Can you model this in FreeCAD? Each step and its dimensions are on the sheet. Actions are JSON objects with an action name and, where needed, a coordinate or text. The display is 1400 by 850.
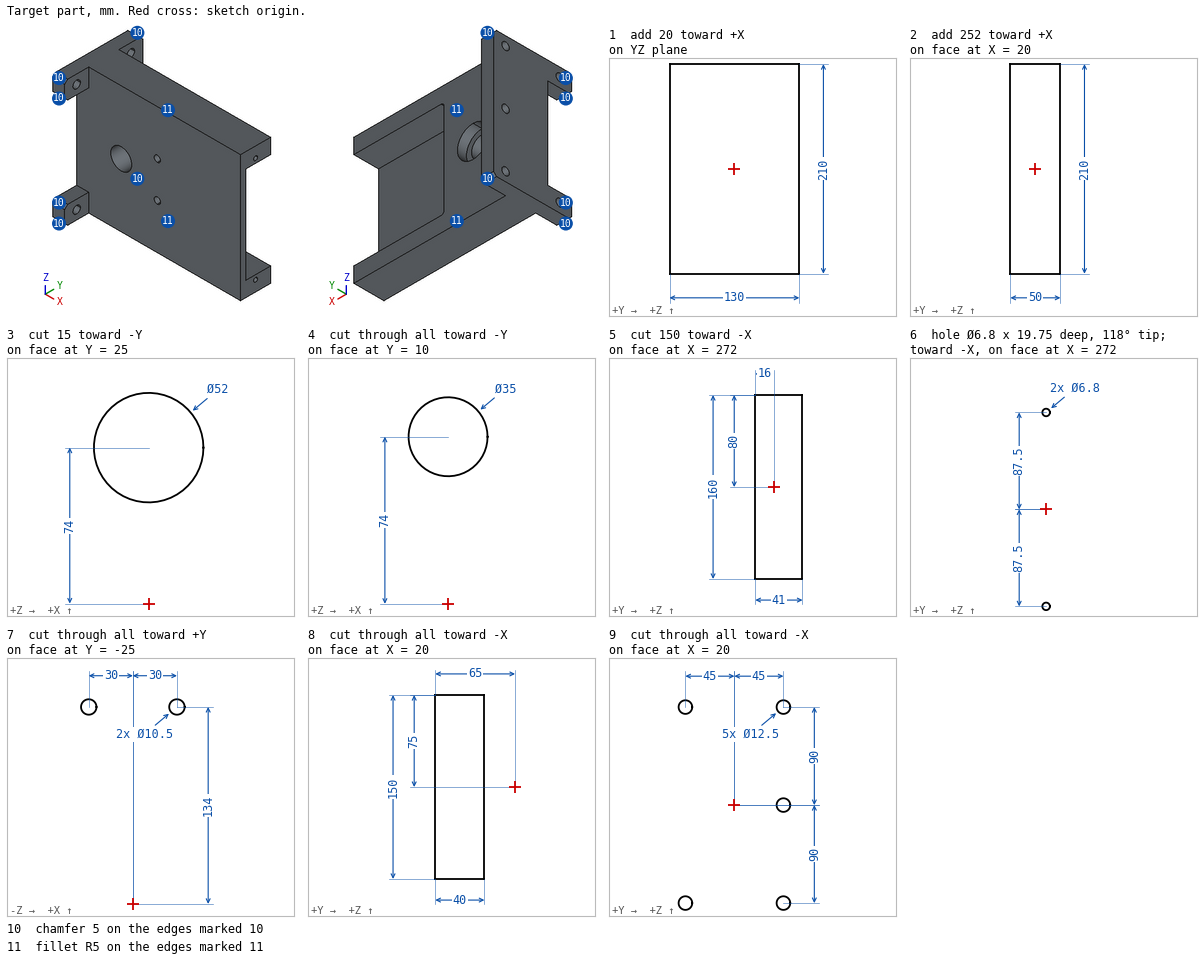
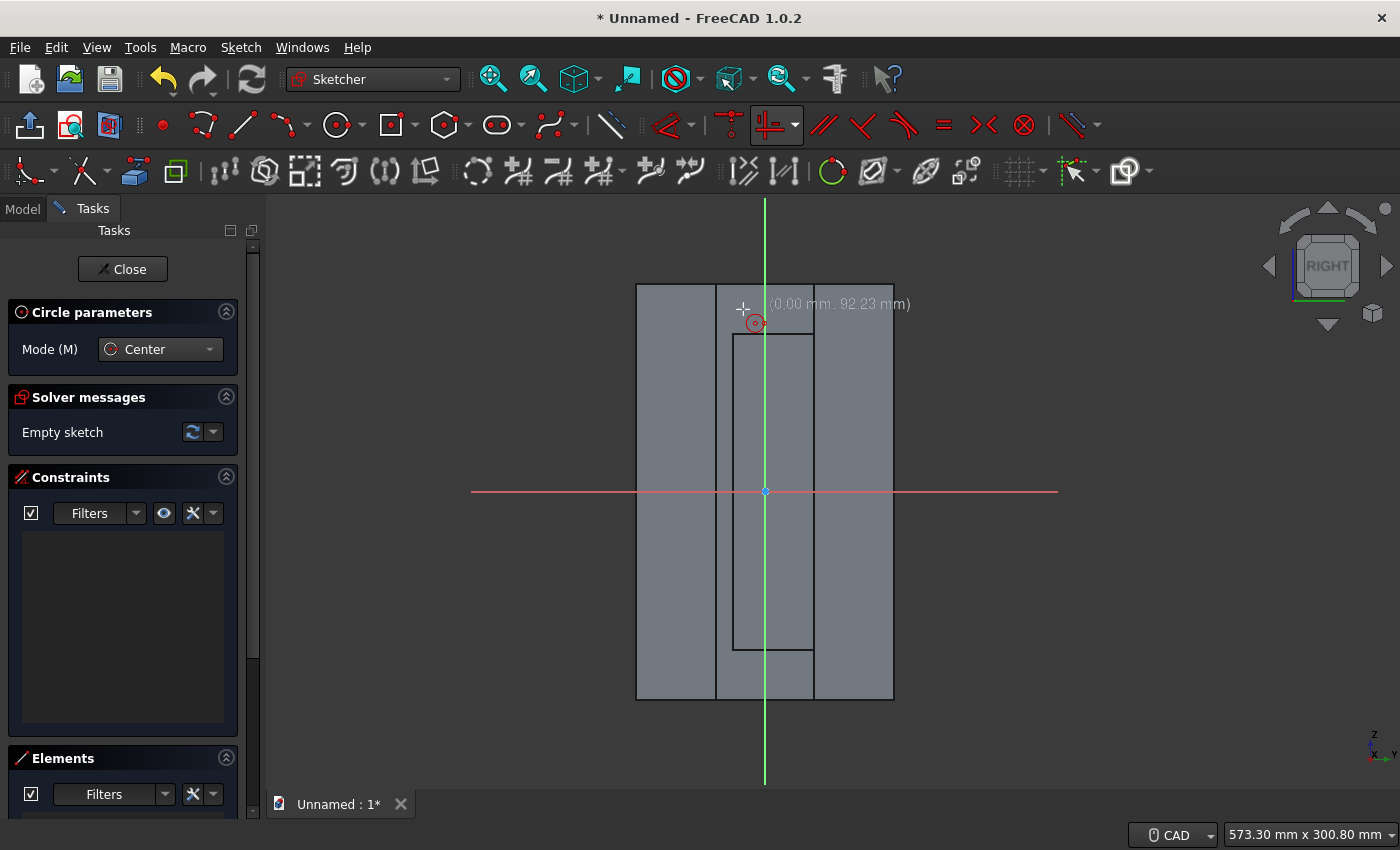
{"action": "left_click", "coordinate": [765, 319]}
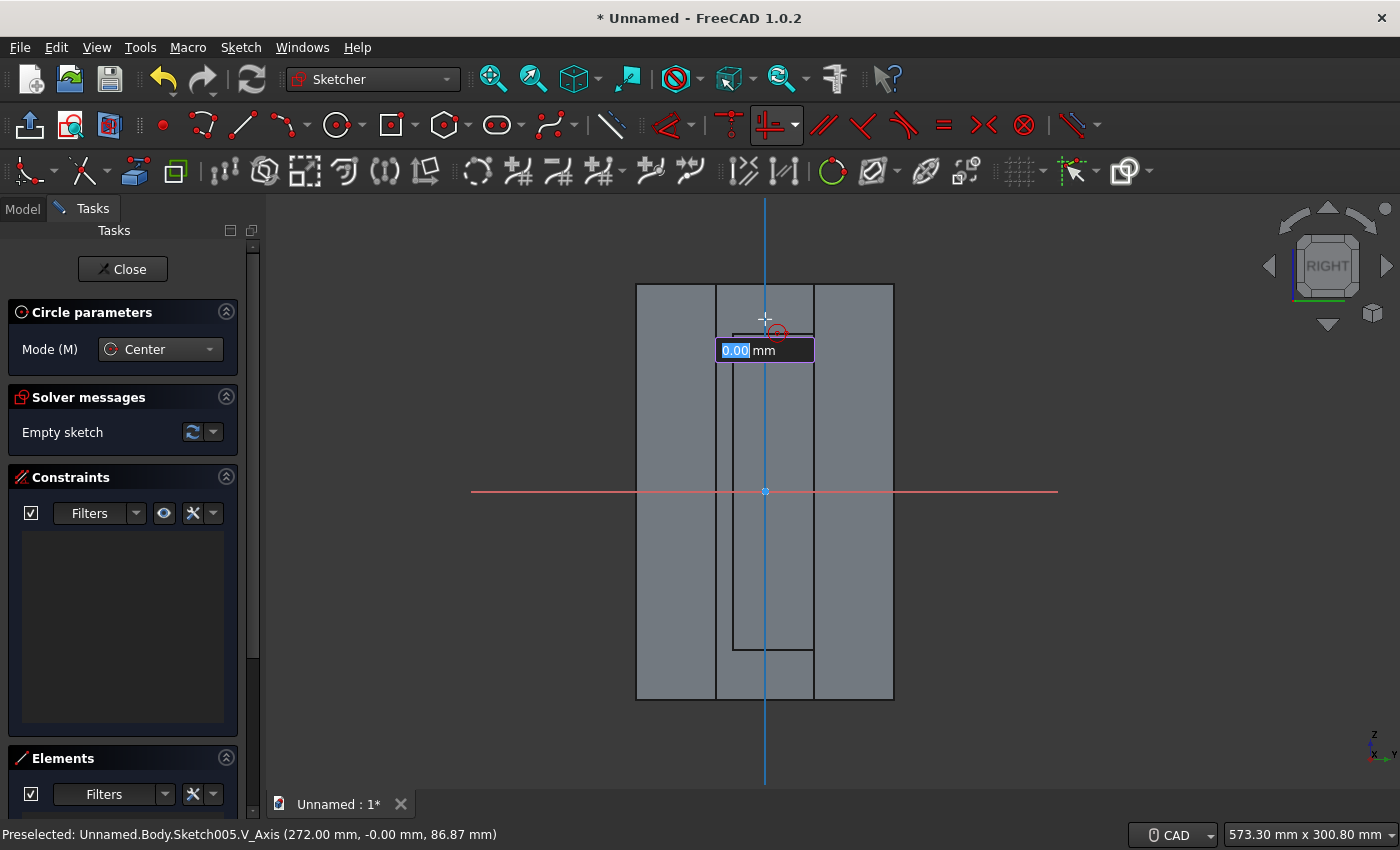
{"action": "scroll", "coordinate": [771, 316], "scroll_direction": "up", "scroll_amount": 5}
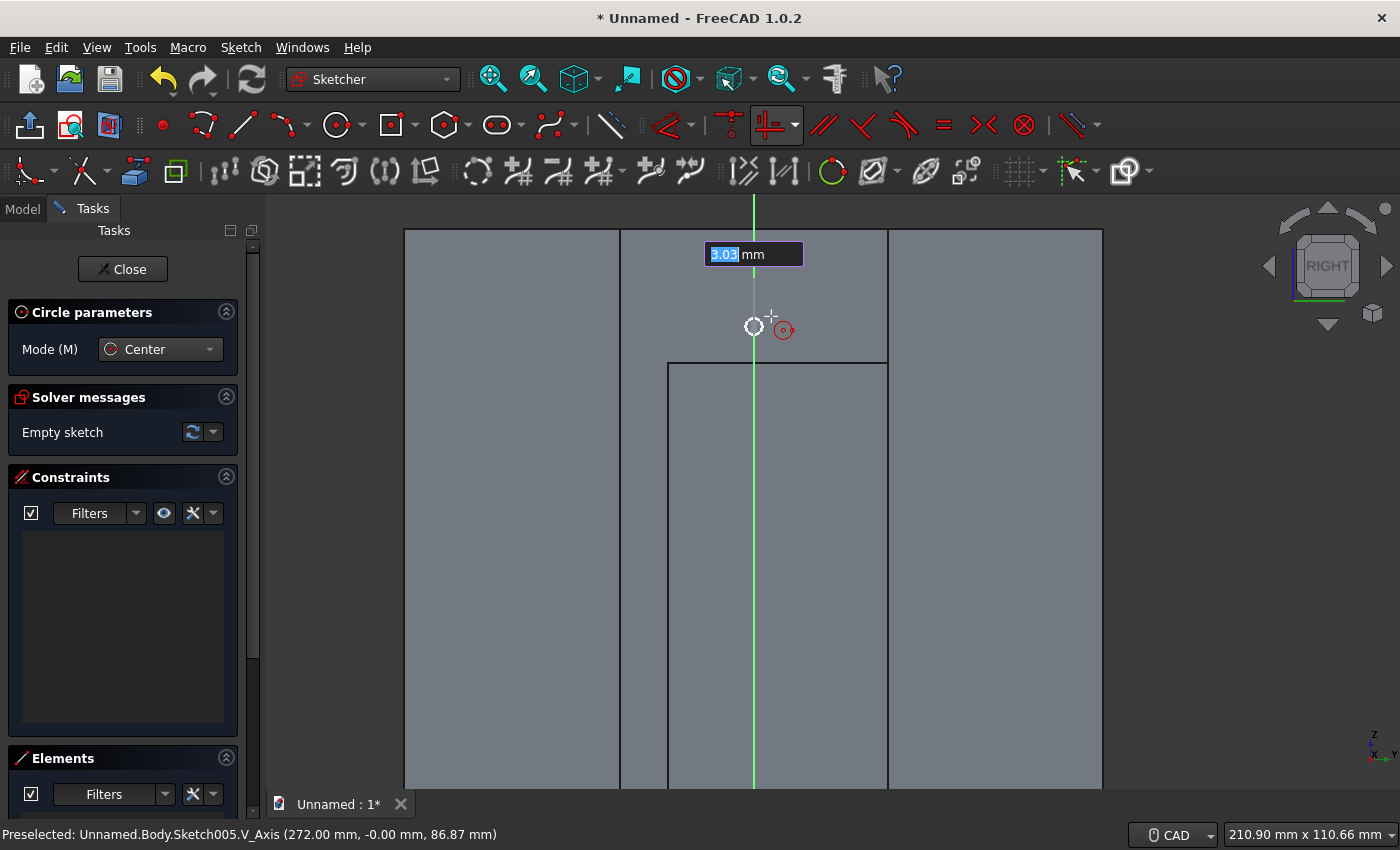
{"action": "left_click", "coordinate": [771, 317]}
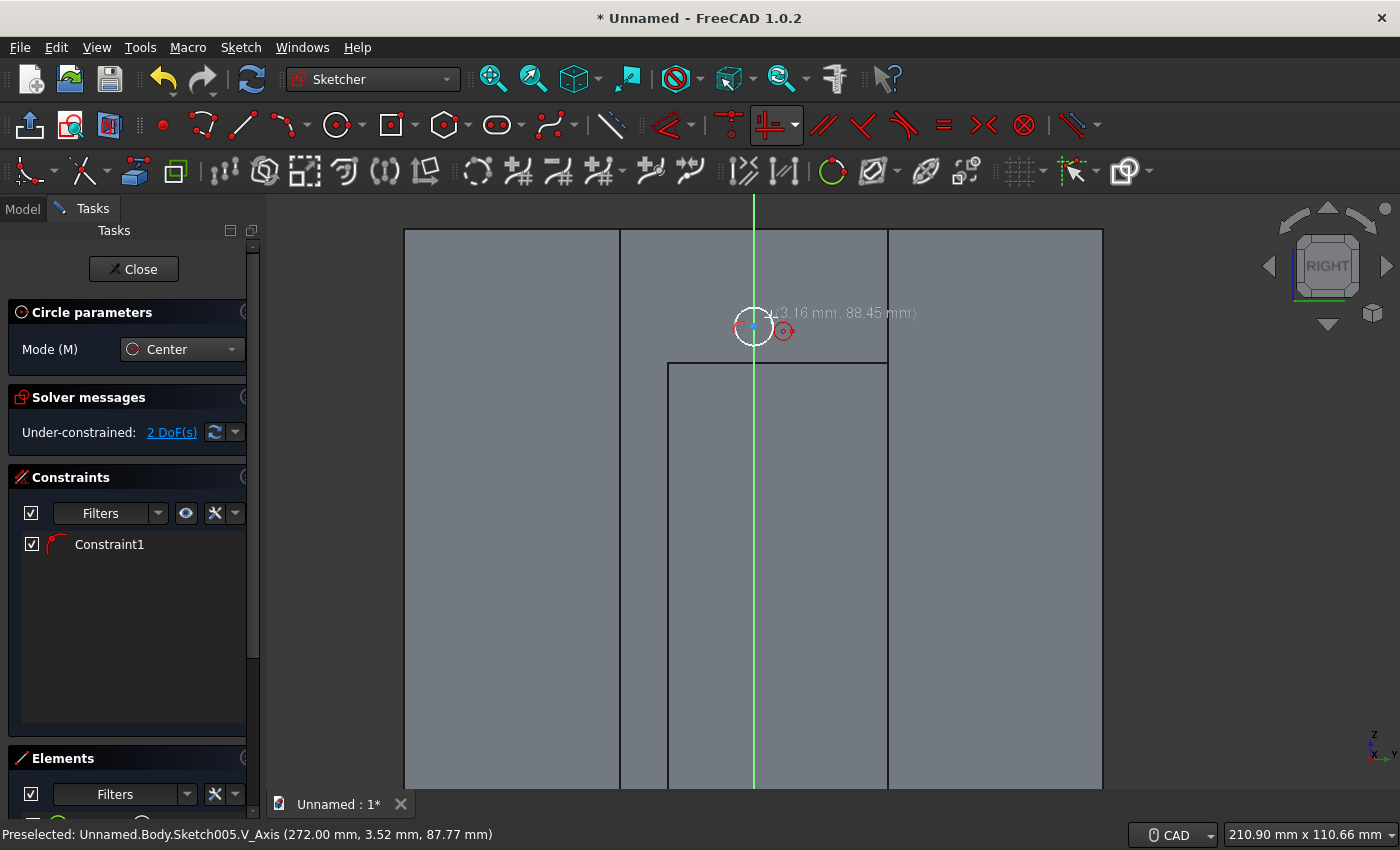
{"action": "scroll", "coordinate": [771, 316], "scroll_direction": "down", "scroll_amount": 5}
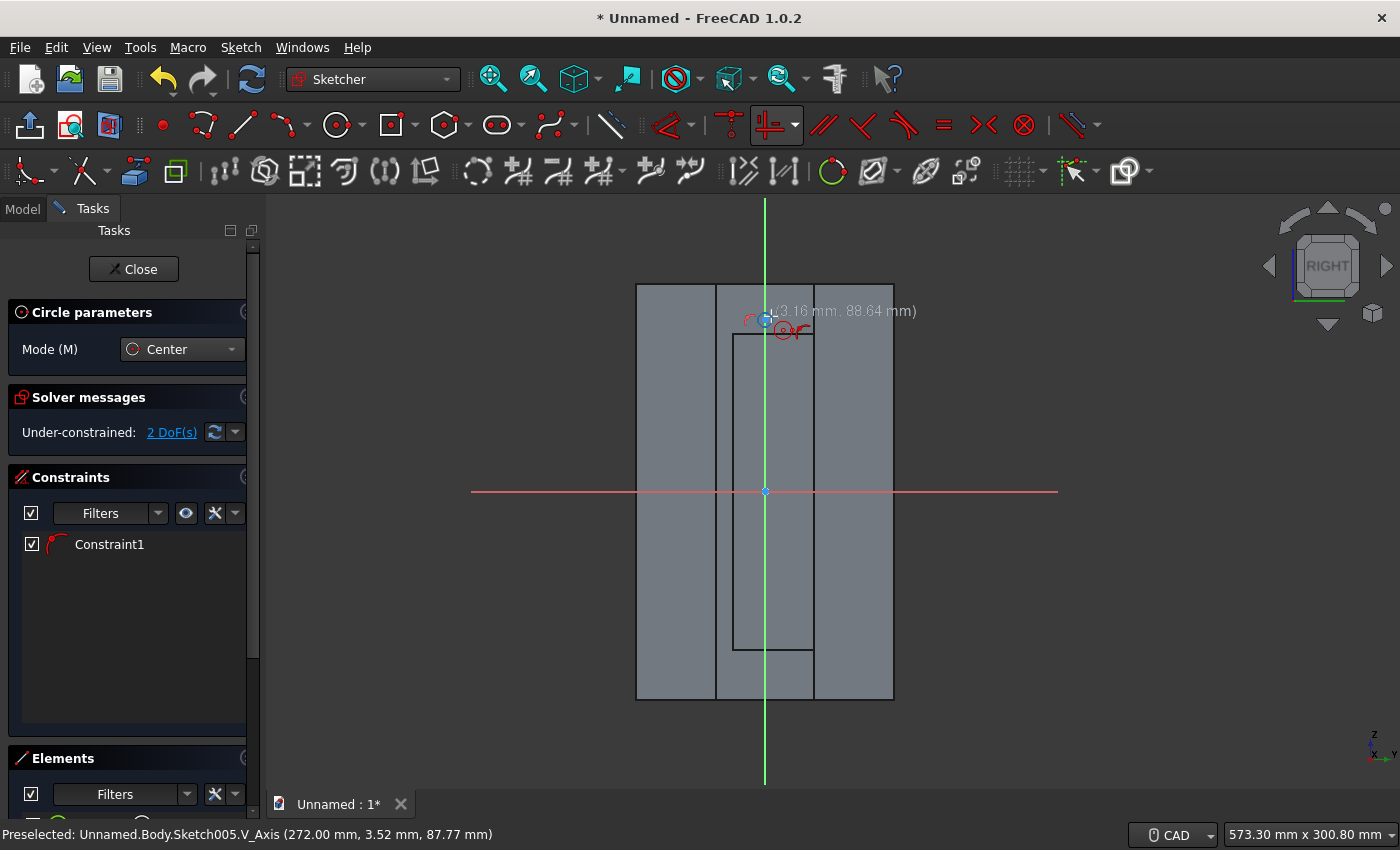
{"action": "scroll", "coordinate": [765, 665], "scroll_direction": "up", "scroll_amount": 7}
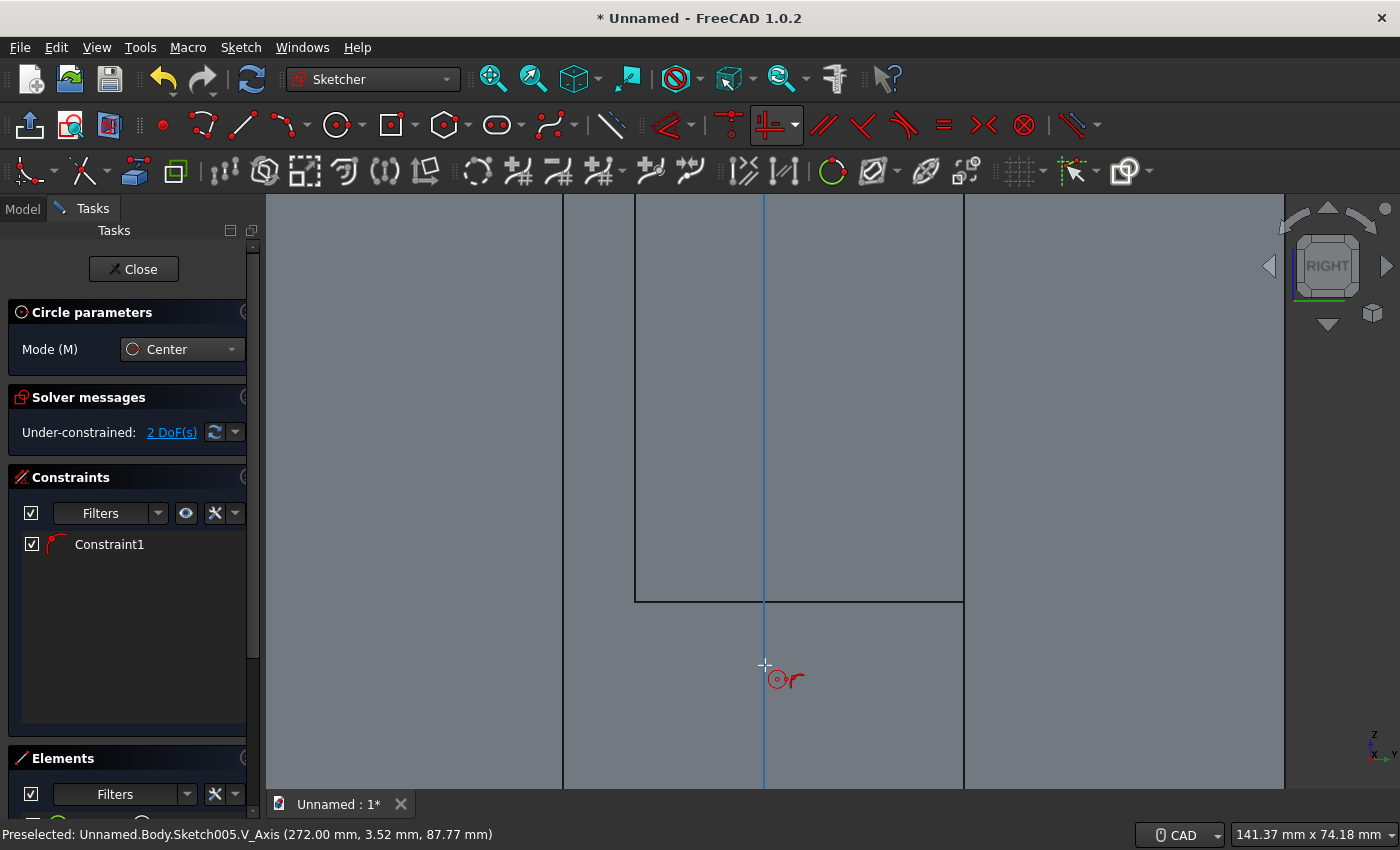
{"action": "scroll", "coordinate": [765, 665], "scroll_direction": "down", "scroll_amount": 7}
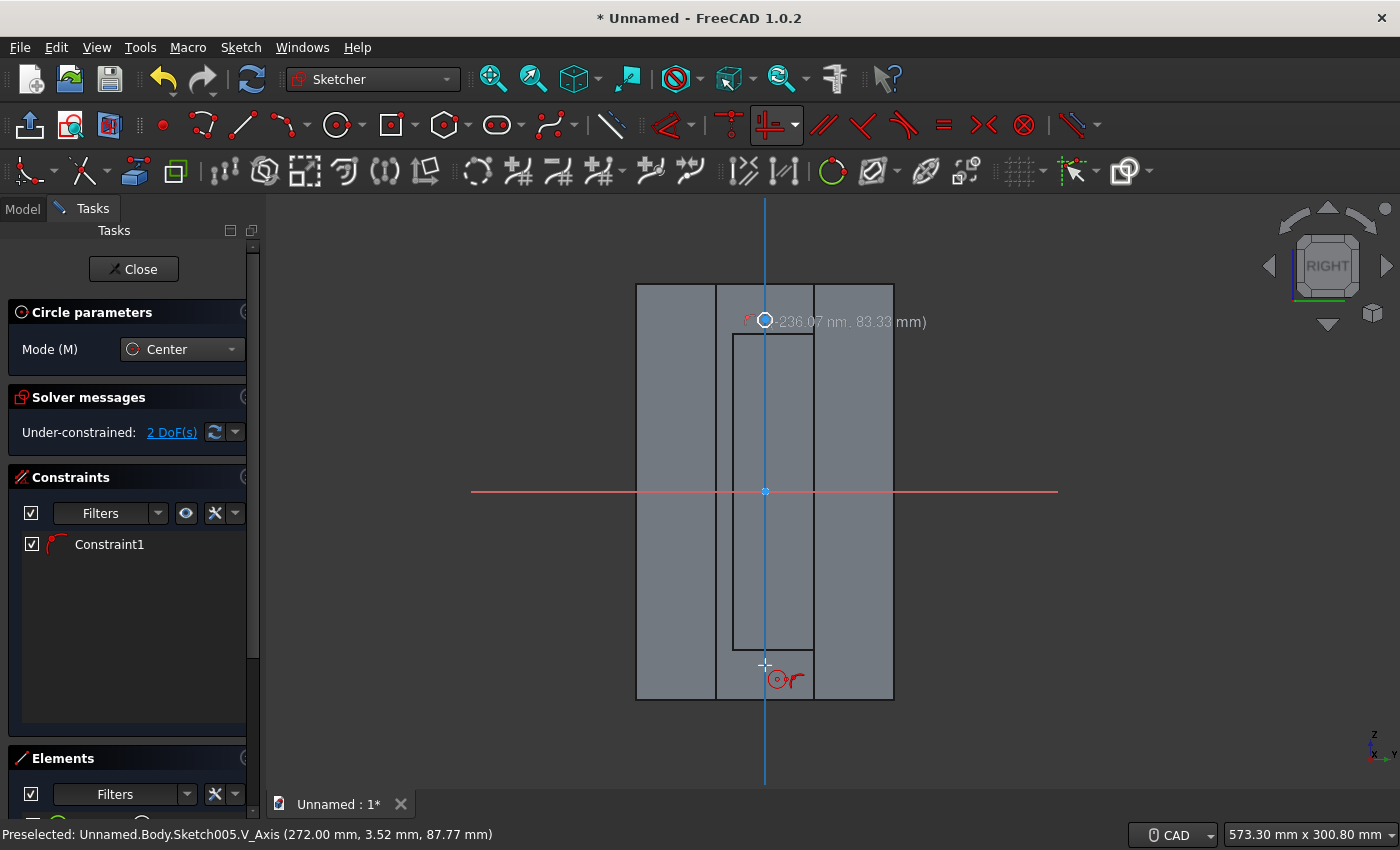
{"action": "left_click", "coordinate": [765, 665]}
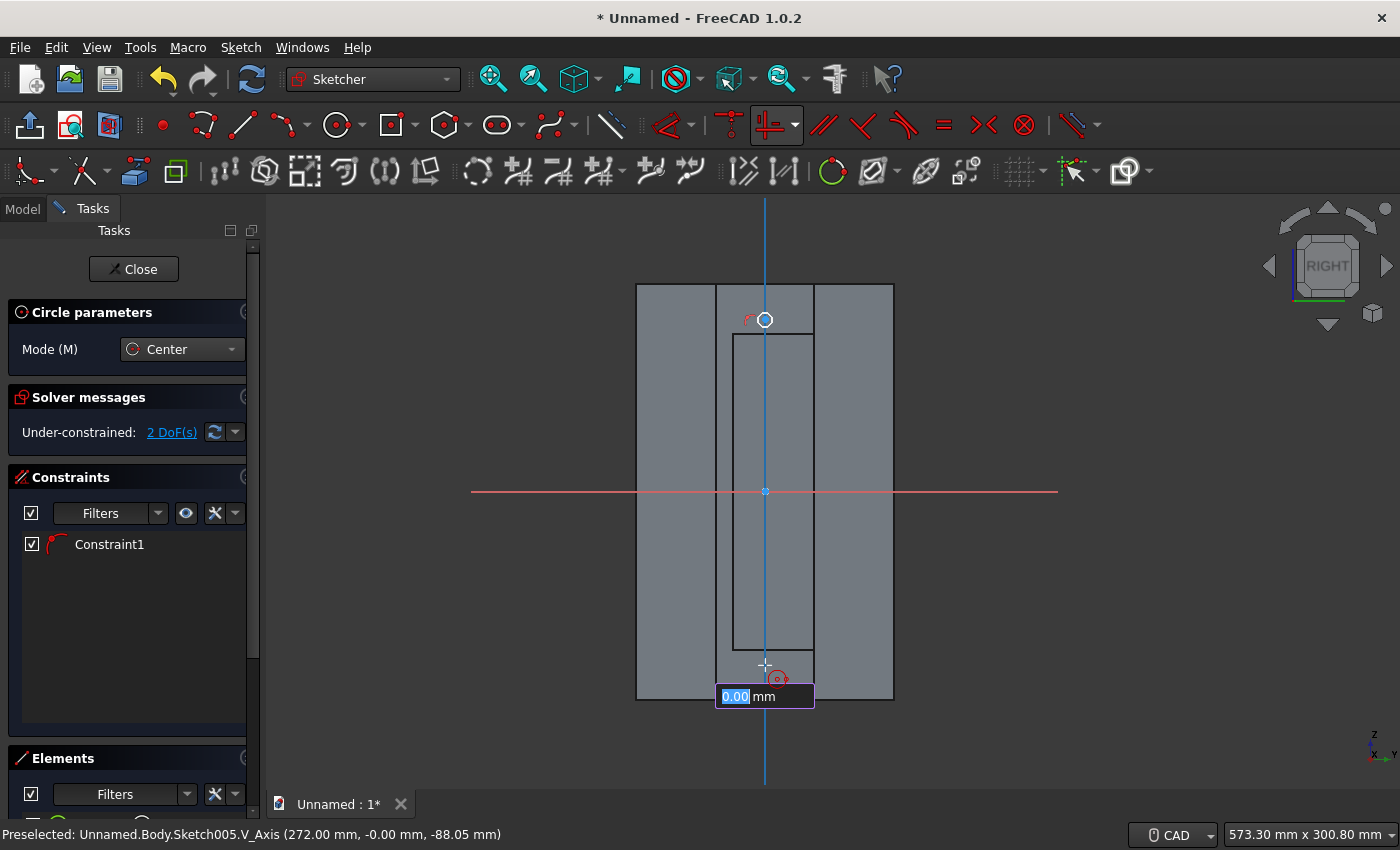
{"action": "scroll", "coordinate": [771, 663], "scroll_direction": "up", "scroll_amount": 5}